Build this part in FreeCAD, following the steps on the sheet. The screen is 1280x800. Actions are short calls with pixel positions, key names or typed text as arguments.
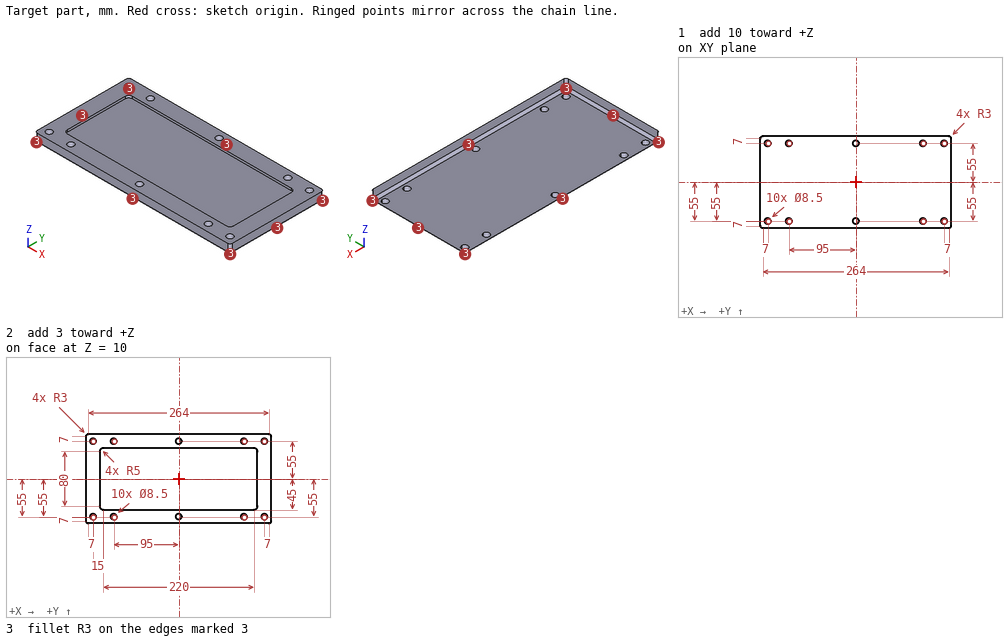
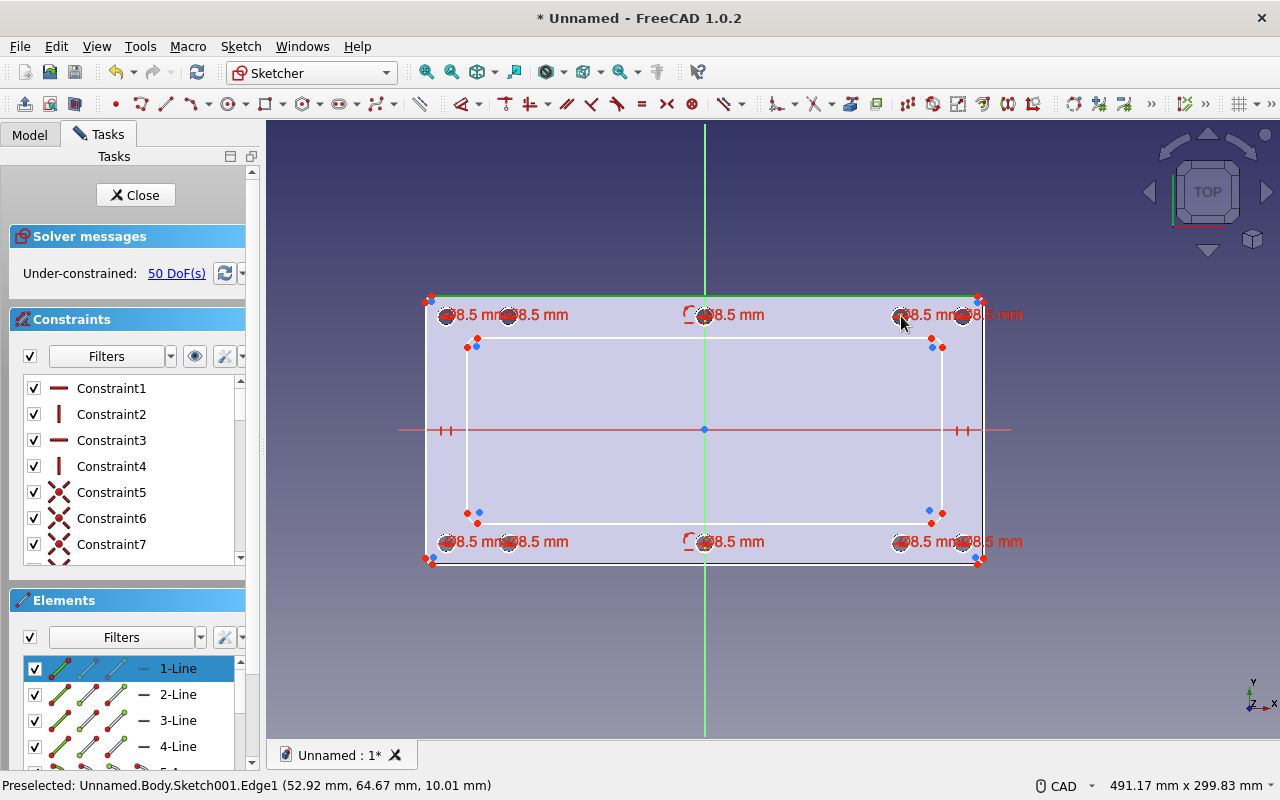
scroll(427, 298, up, 6)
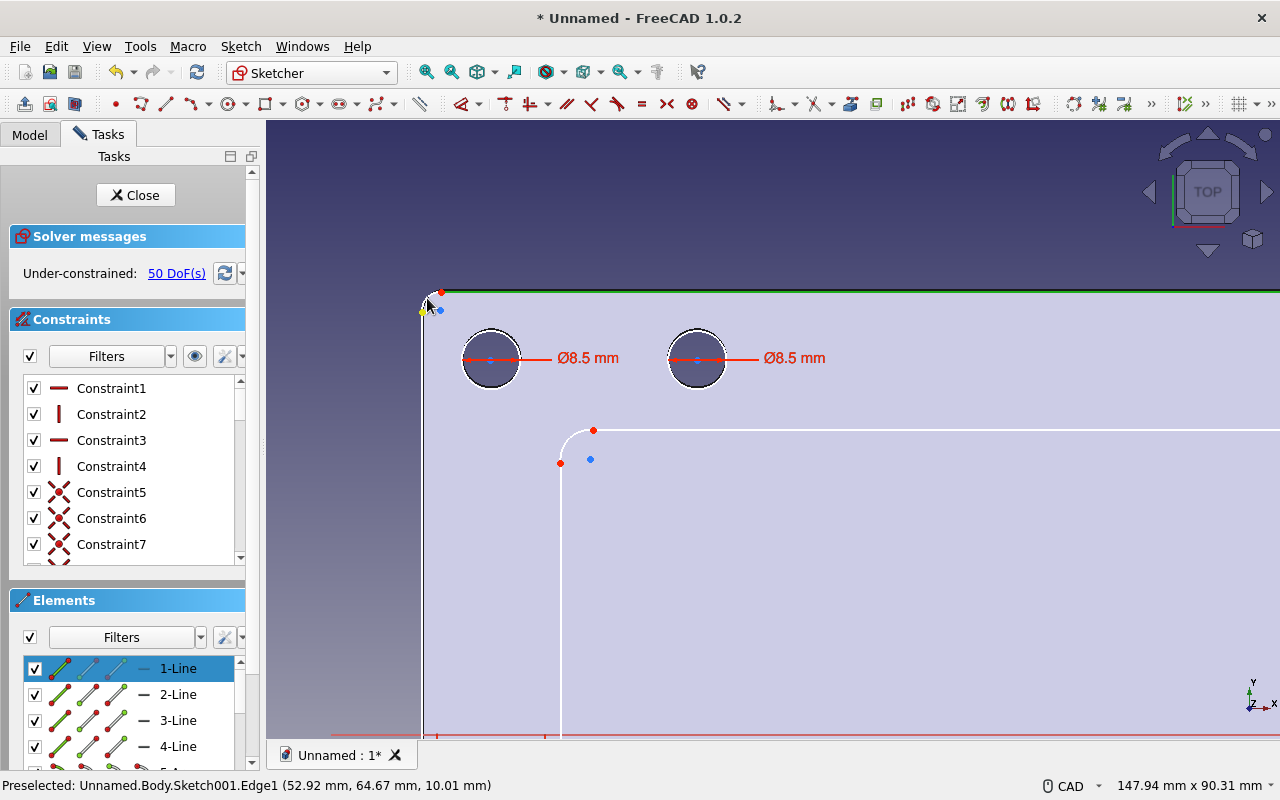
click(427, 298)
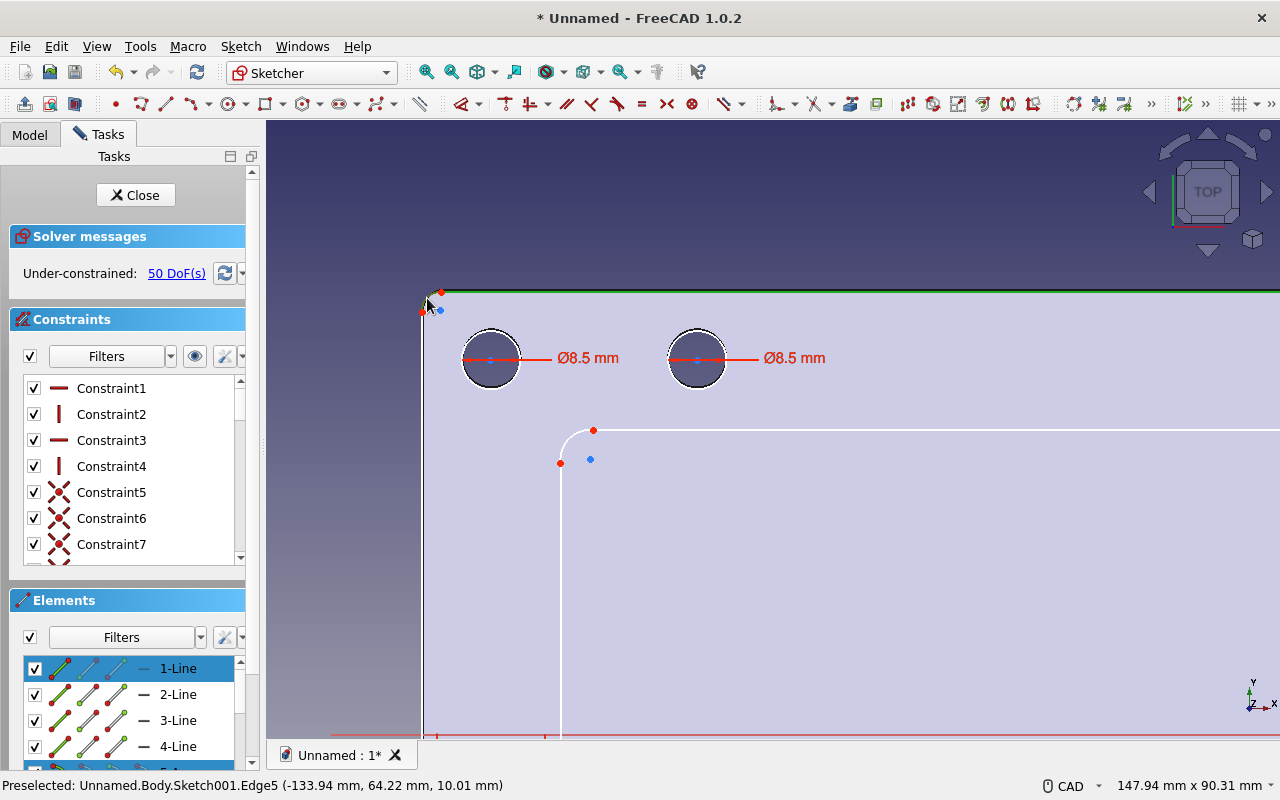
click(617, 104)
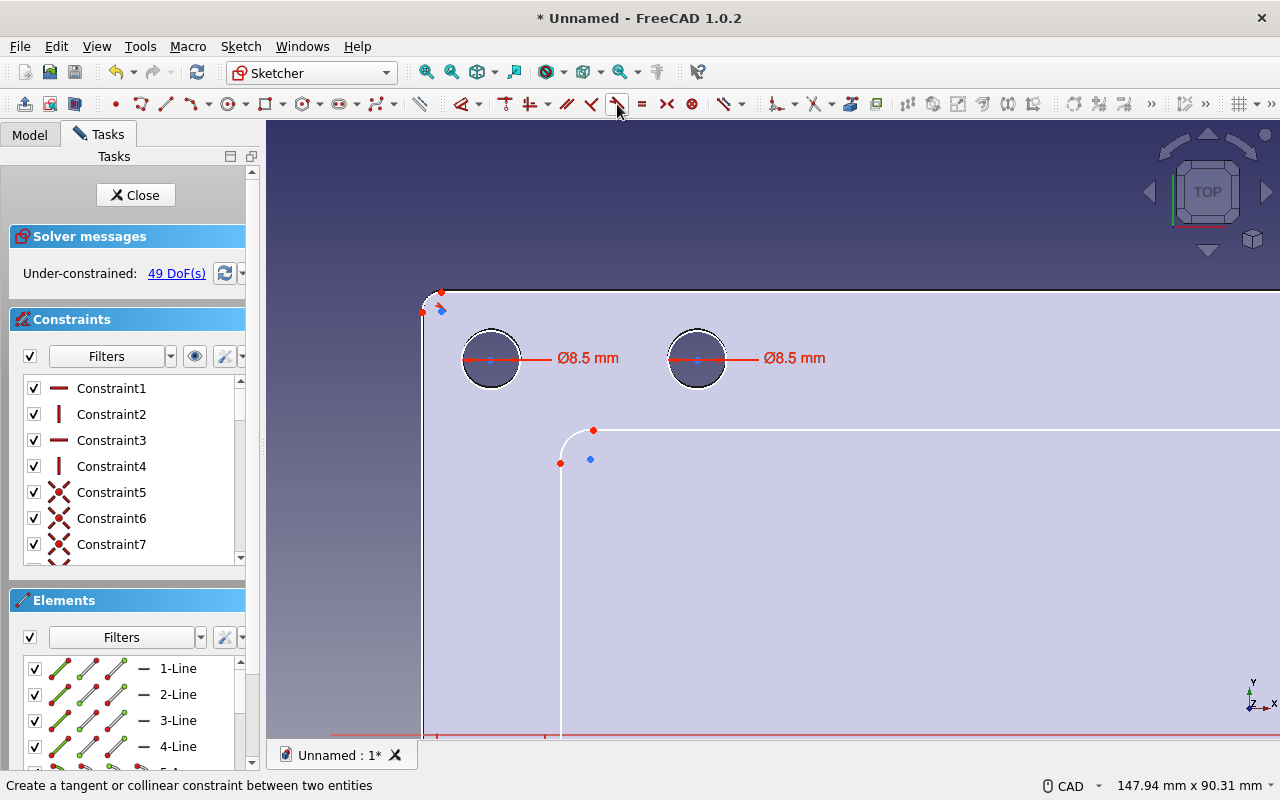
click(986, 292)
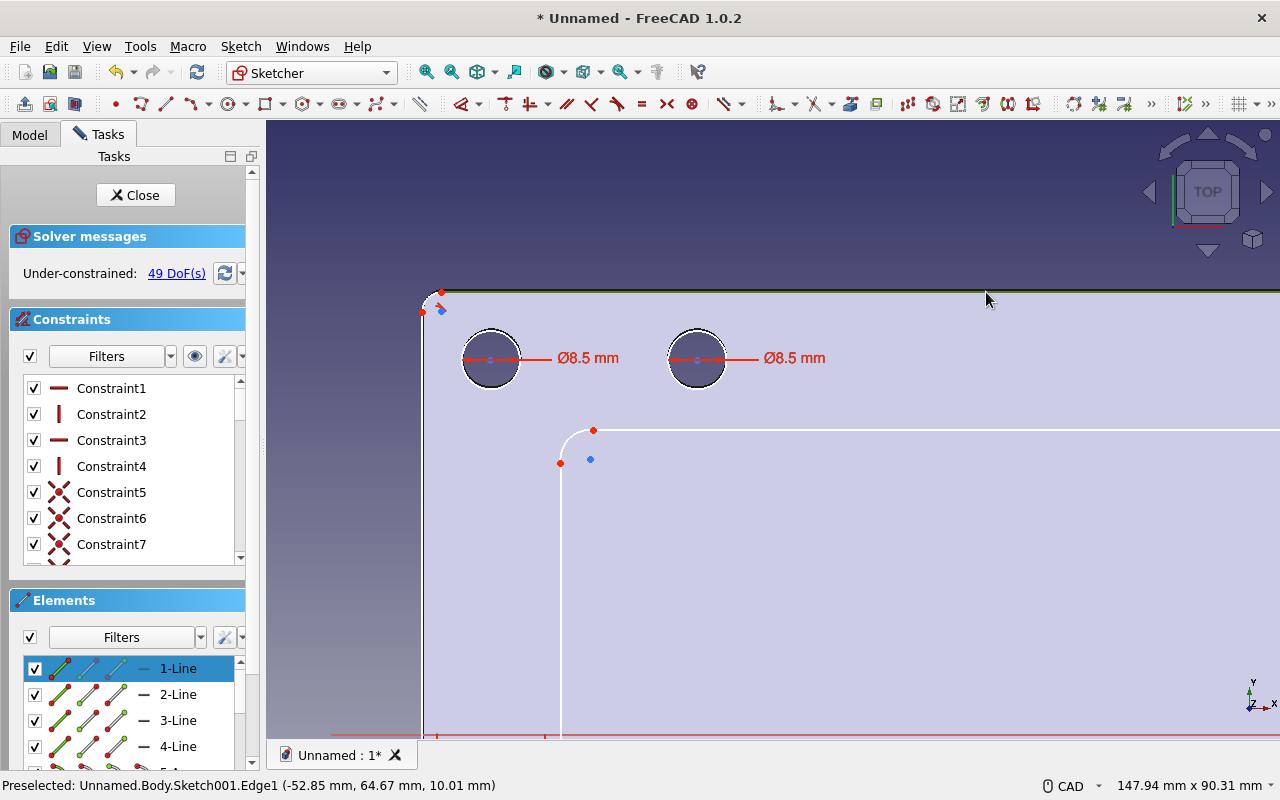
scroll(427, 298, down, 6)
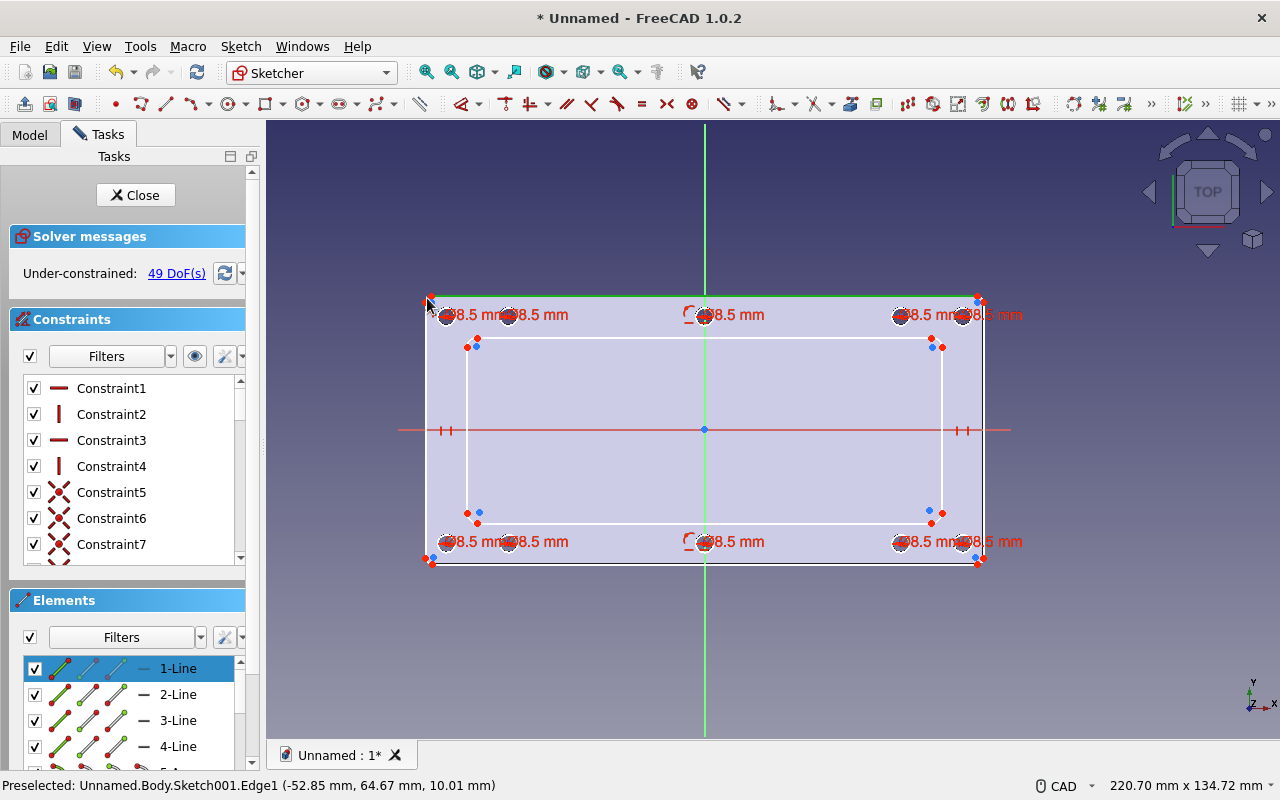
scroll(983, 300, up, 8)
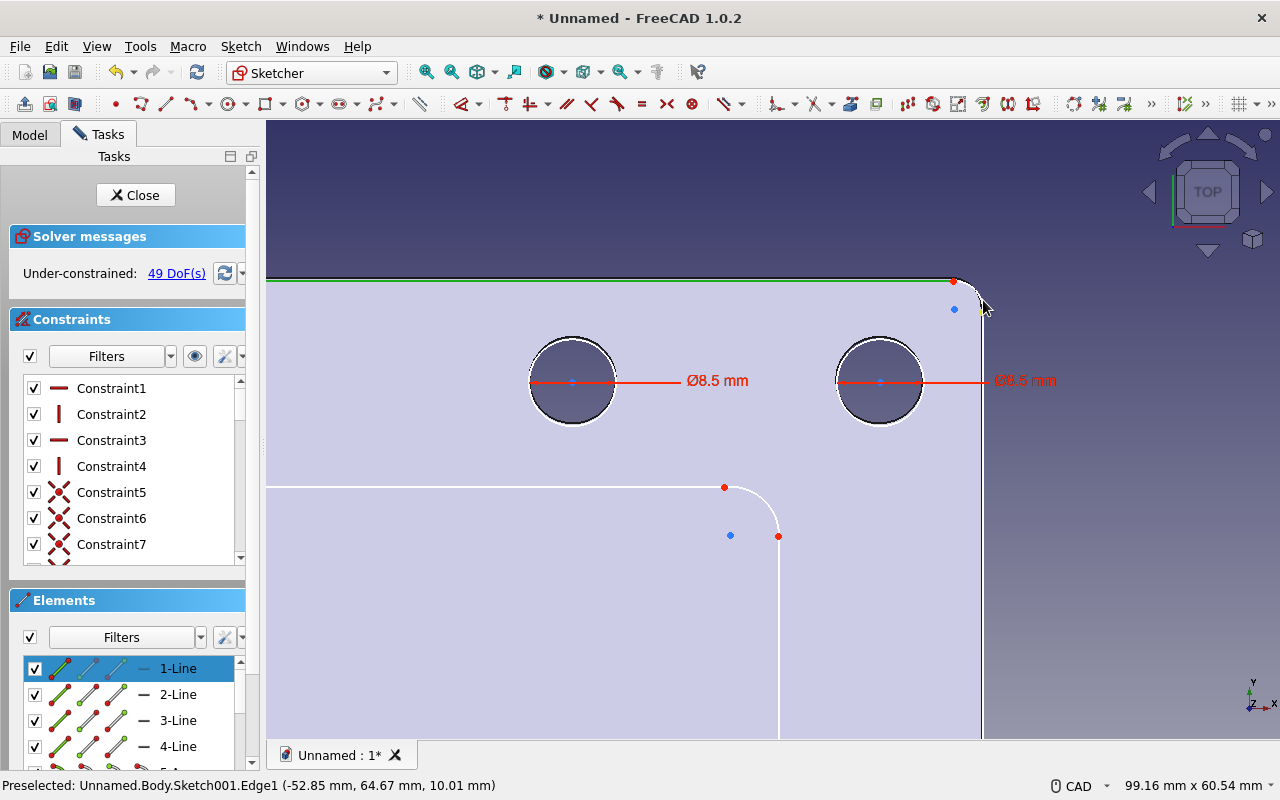
click(981, 298)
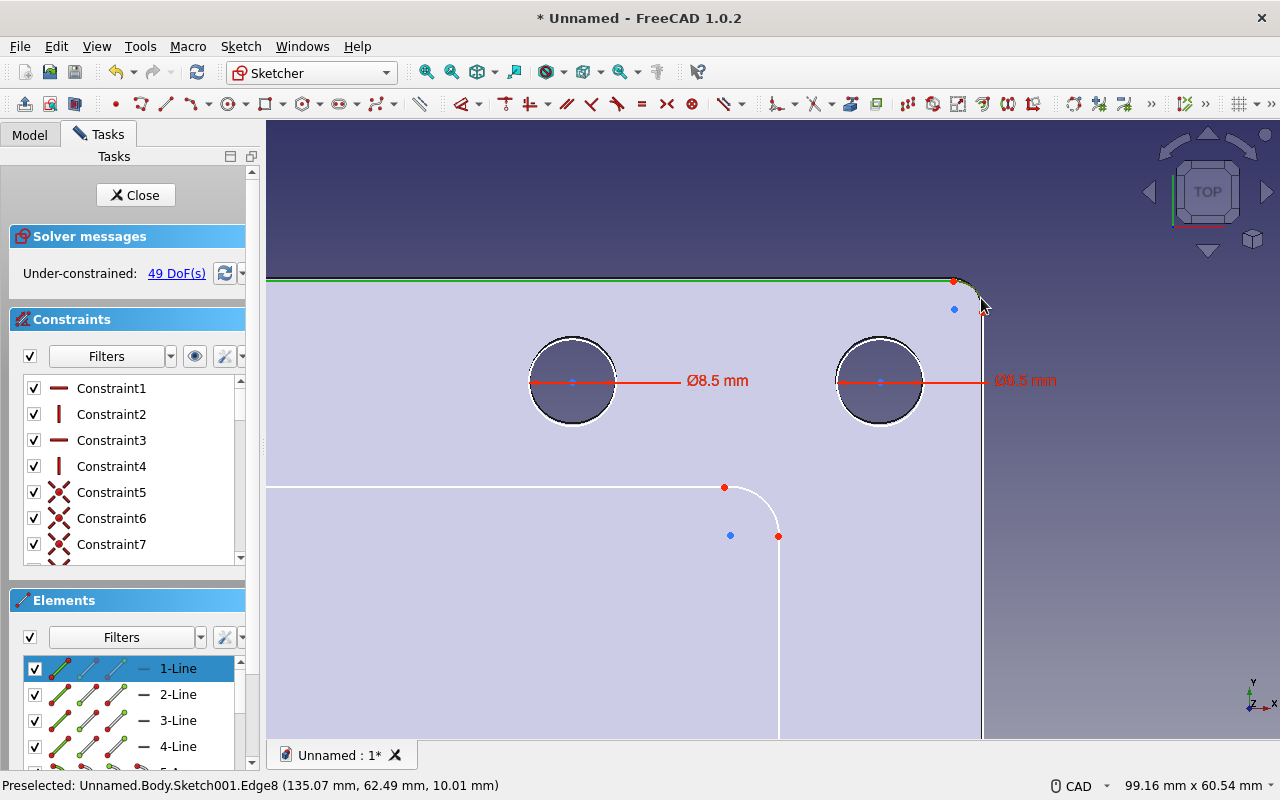
click(617, 104)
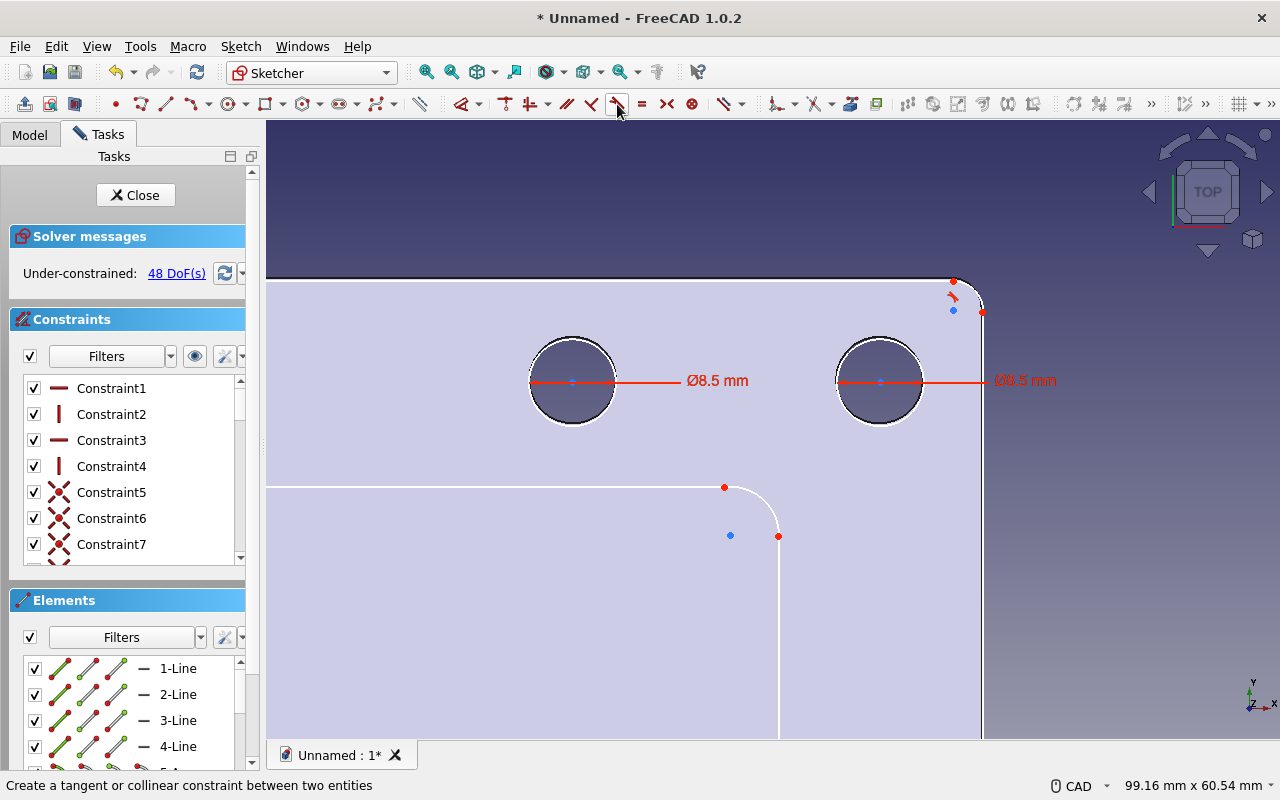
scroll(984, 300, down, 8)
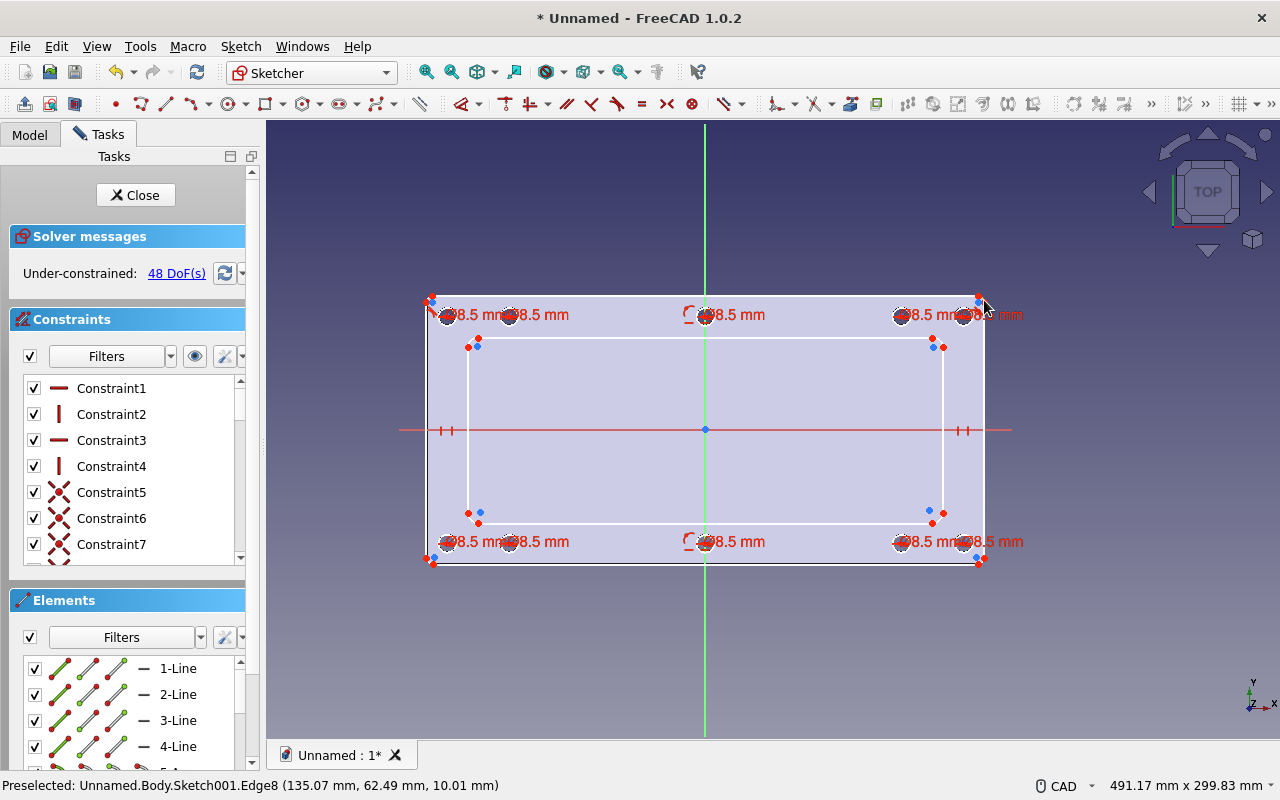
click(426, 379)